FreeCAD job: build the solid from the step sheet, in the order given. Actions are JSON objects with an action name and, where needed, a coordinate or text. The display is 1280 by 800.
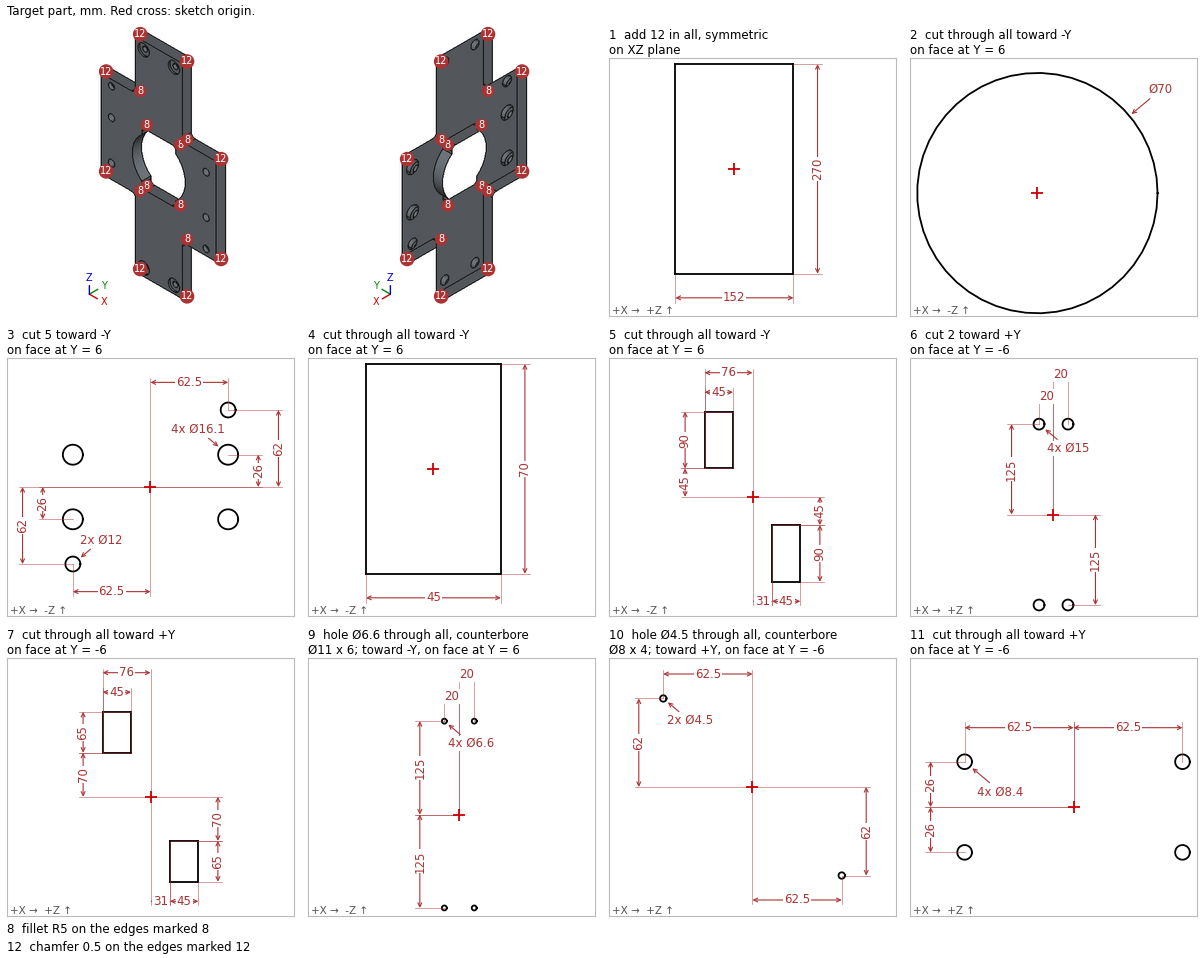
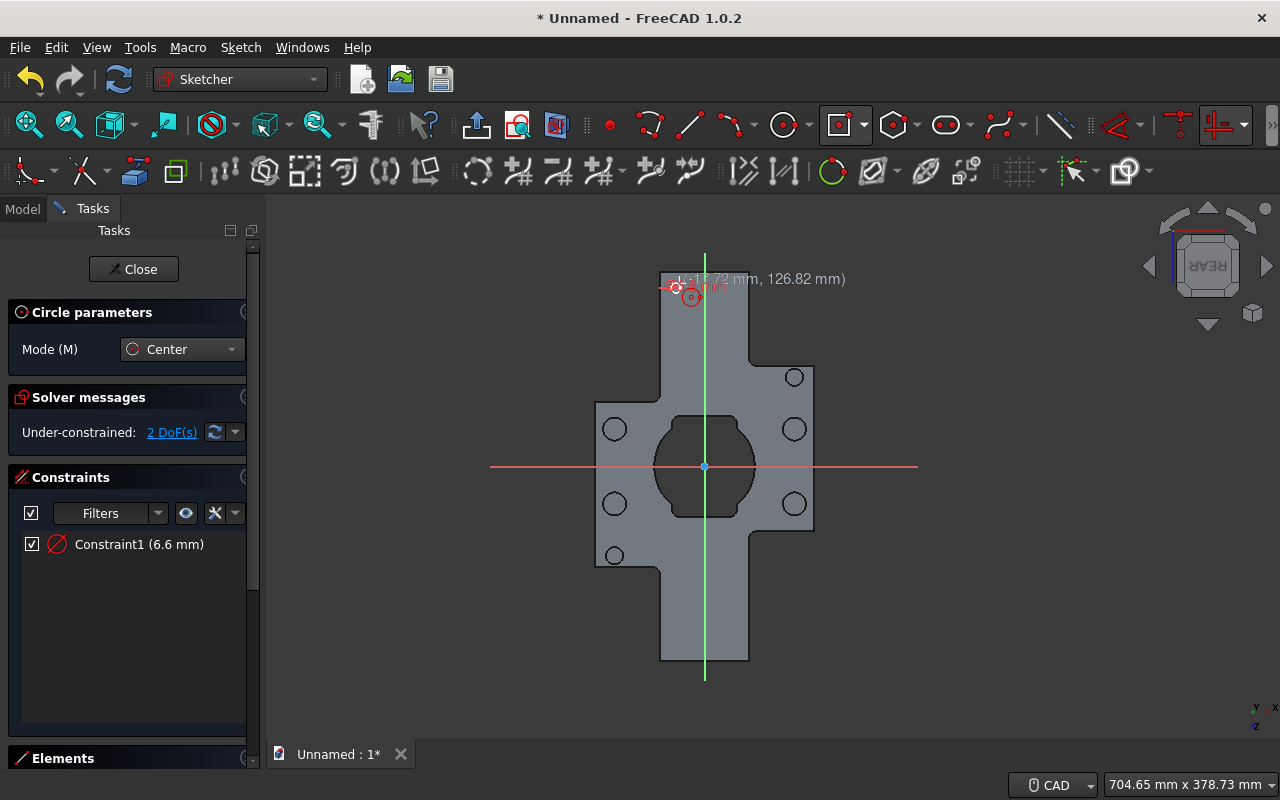
{"action": "scroll", "coordinate": [733, 287], "scroll_direction": "up", "scroll_amount": 8}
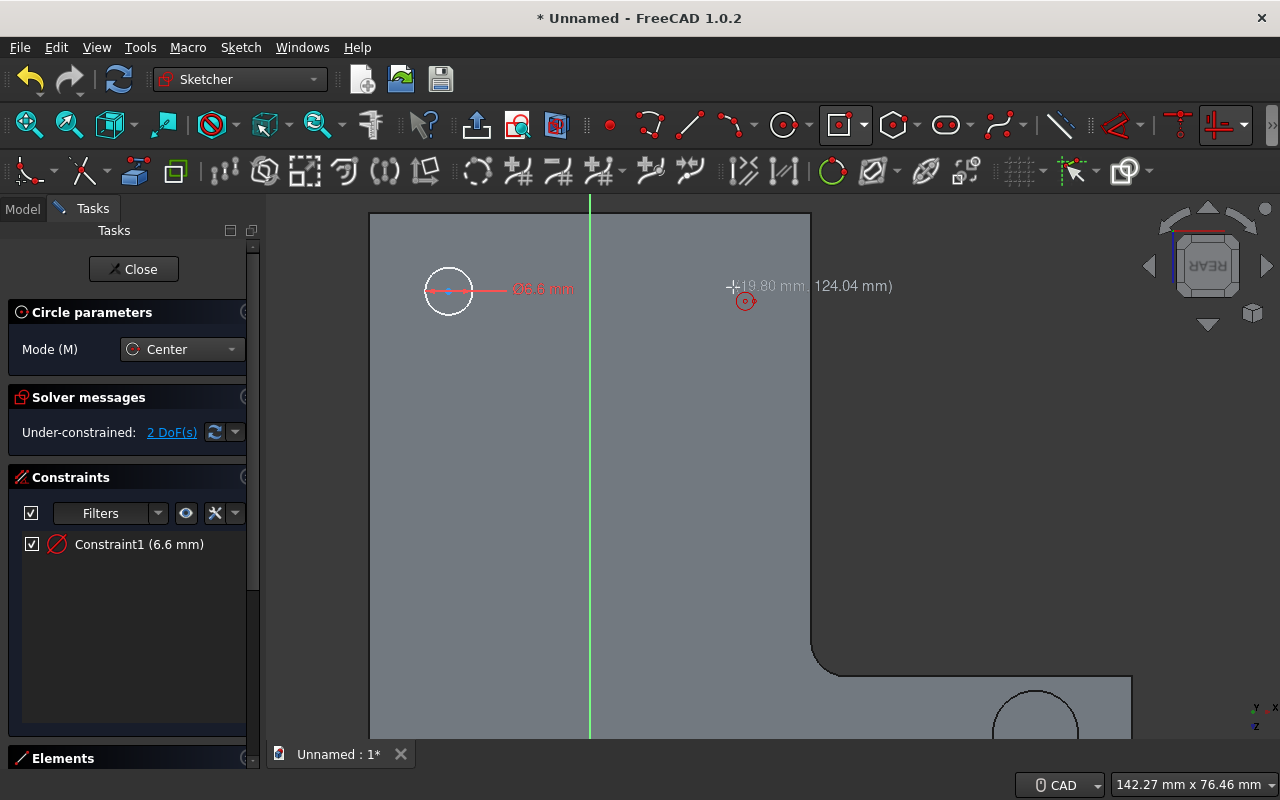
{"action": "scroll", "coordinate": [733, 287], "scroll_direction": "down", "scroll_amount": 8}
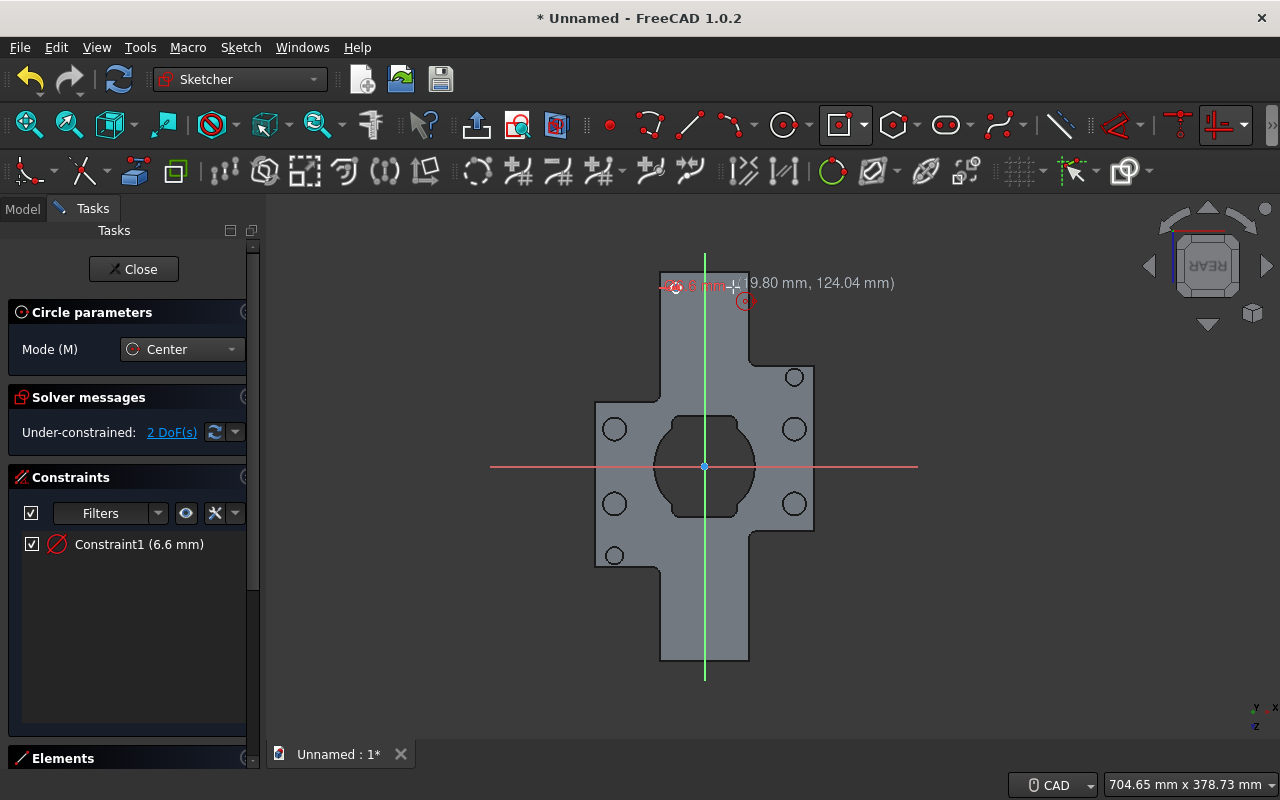
{"action": "left_click", "coordinate": [733, 287]}
{"action": "mouse_move", "coordinate": [737, 283]}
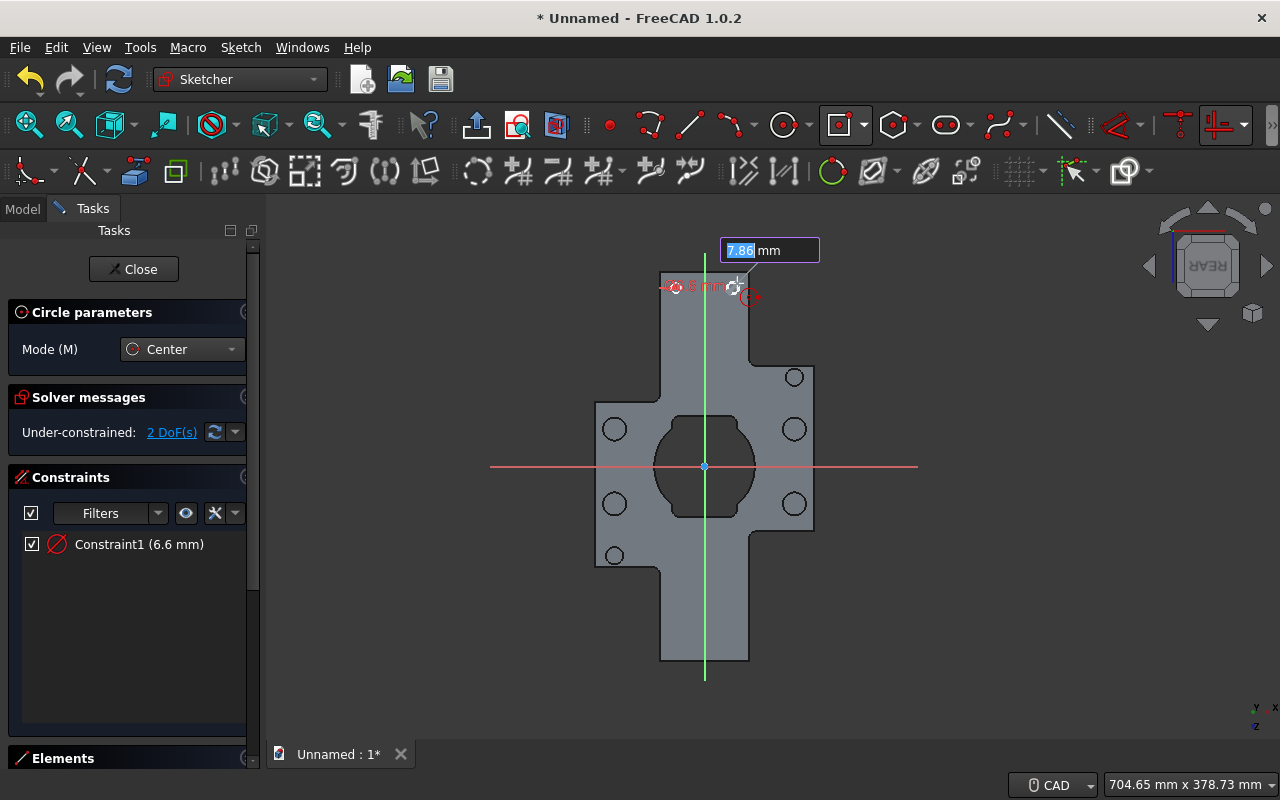
{"action": "type", "text": "6.6"}
{"action": "key", "text": "Return"}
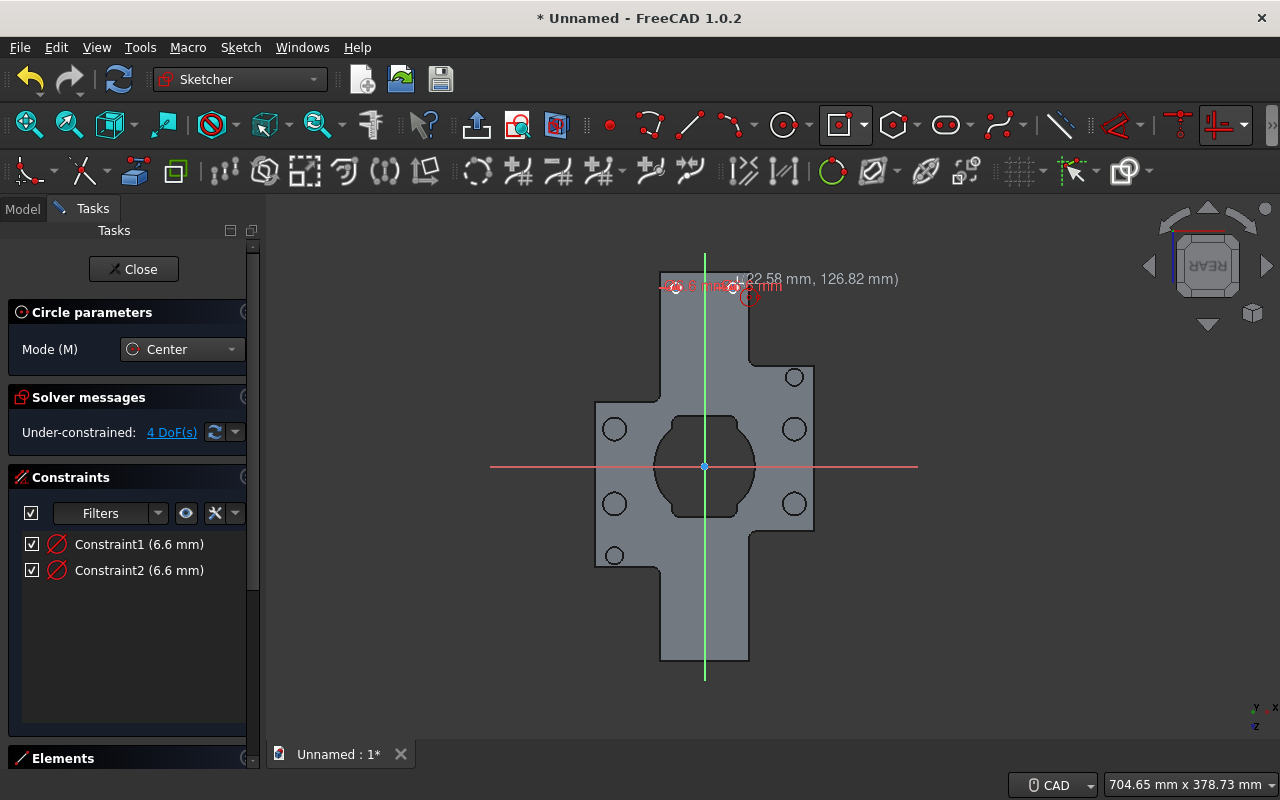
{"action": "scroll", "coordinate": [676, 646], "scroll_direction": "up", "scroll_amount": 8}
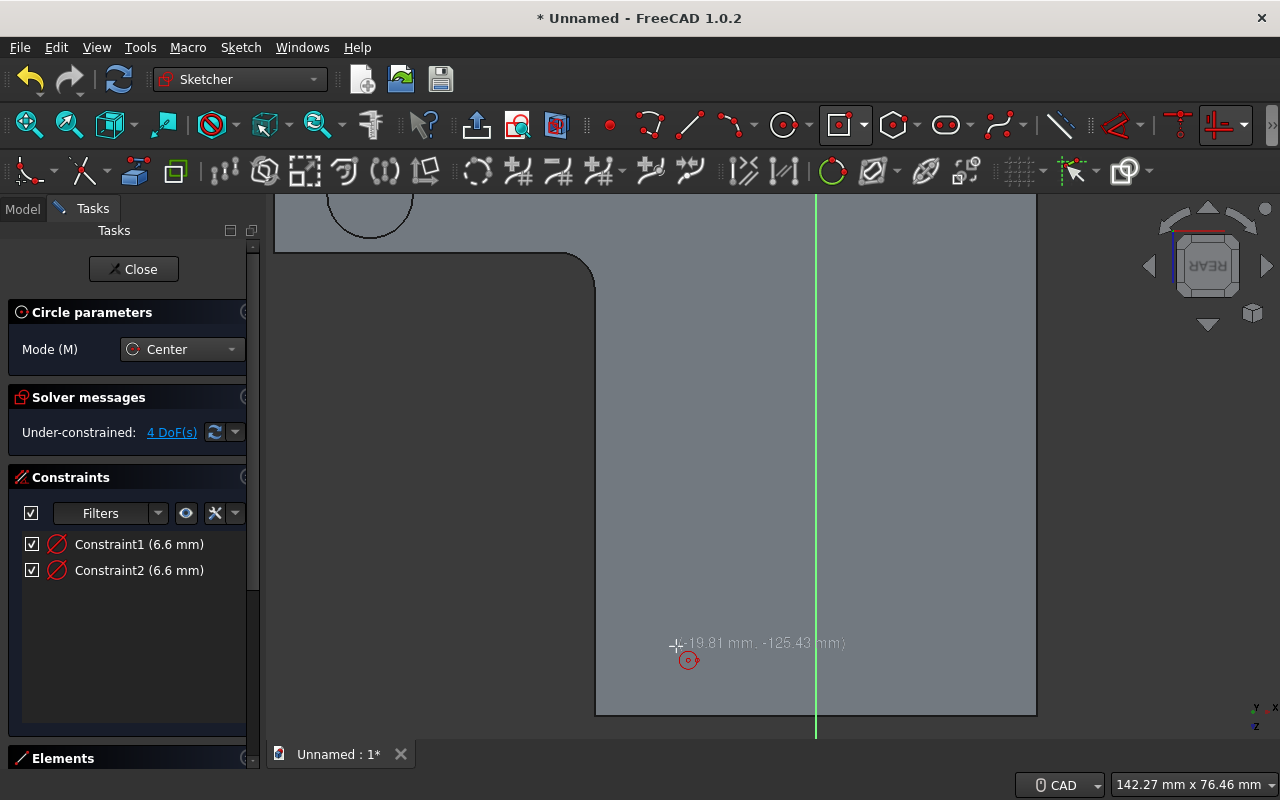
{"action": "scroll", "coordinate": [676, 647], "scroll_direction": "down", "scroll_amount": 8}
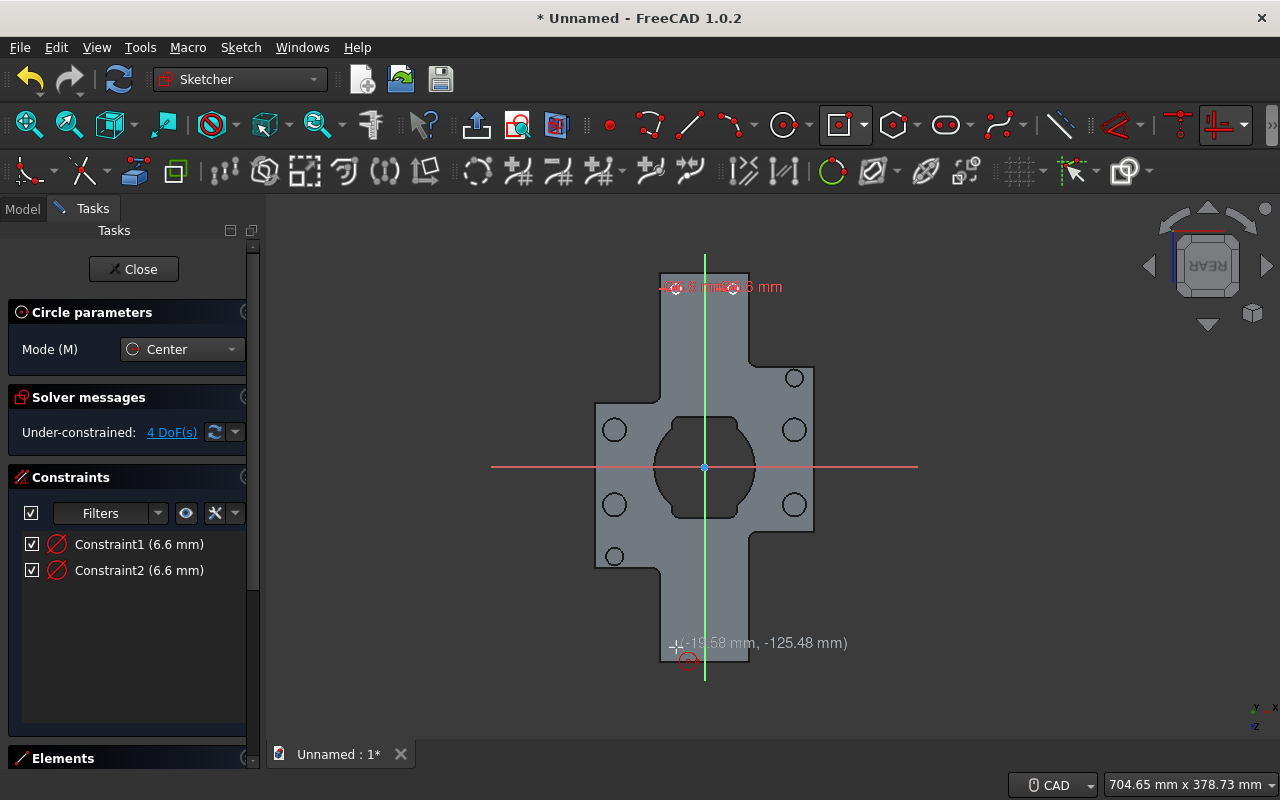
{"action": "left_click", "coordinate": [676, 647]}
{"action": "mouse_move", "coordinate": [679, 644]}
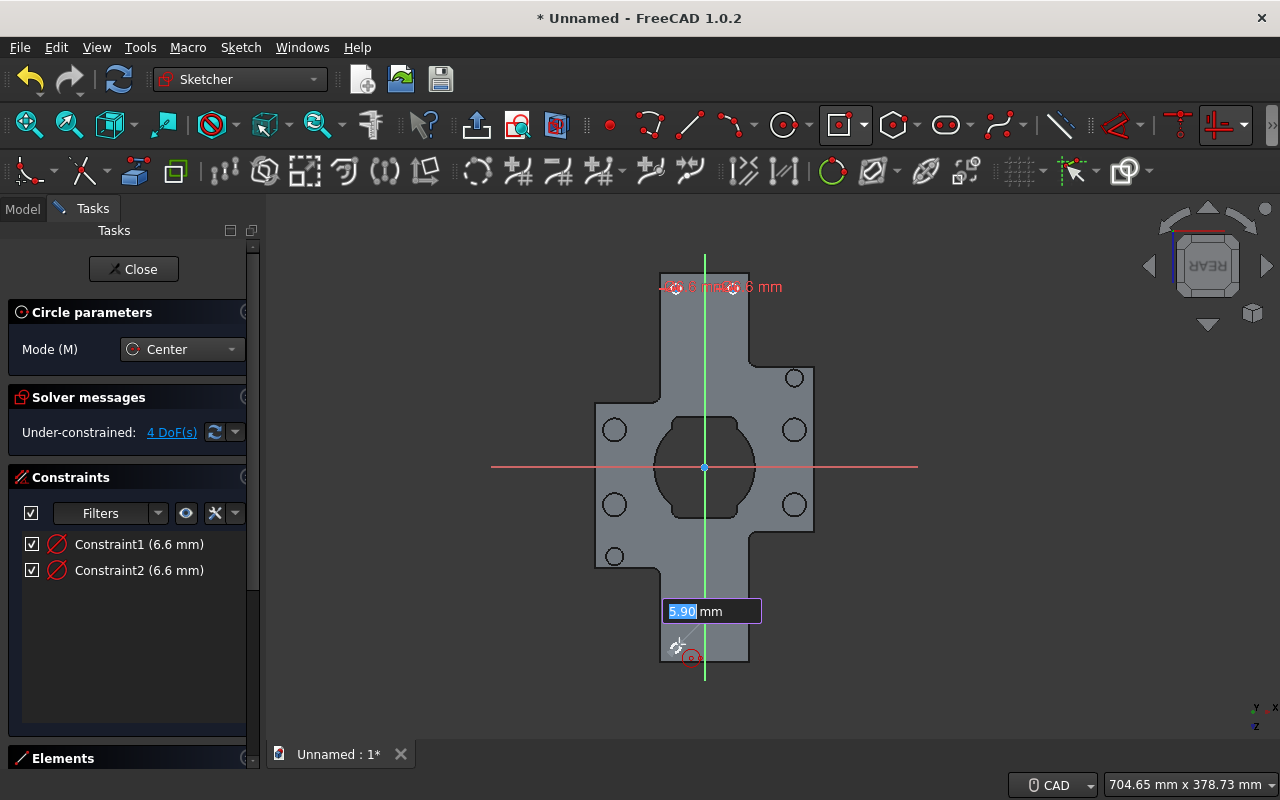
{"action": "type", "text": "6.6"}
{"action": "key", "text": "Return"}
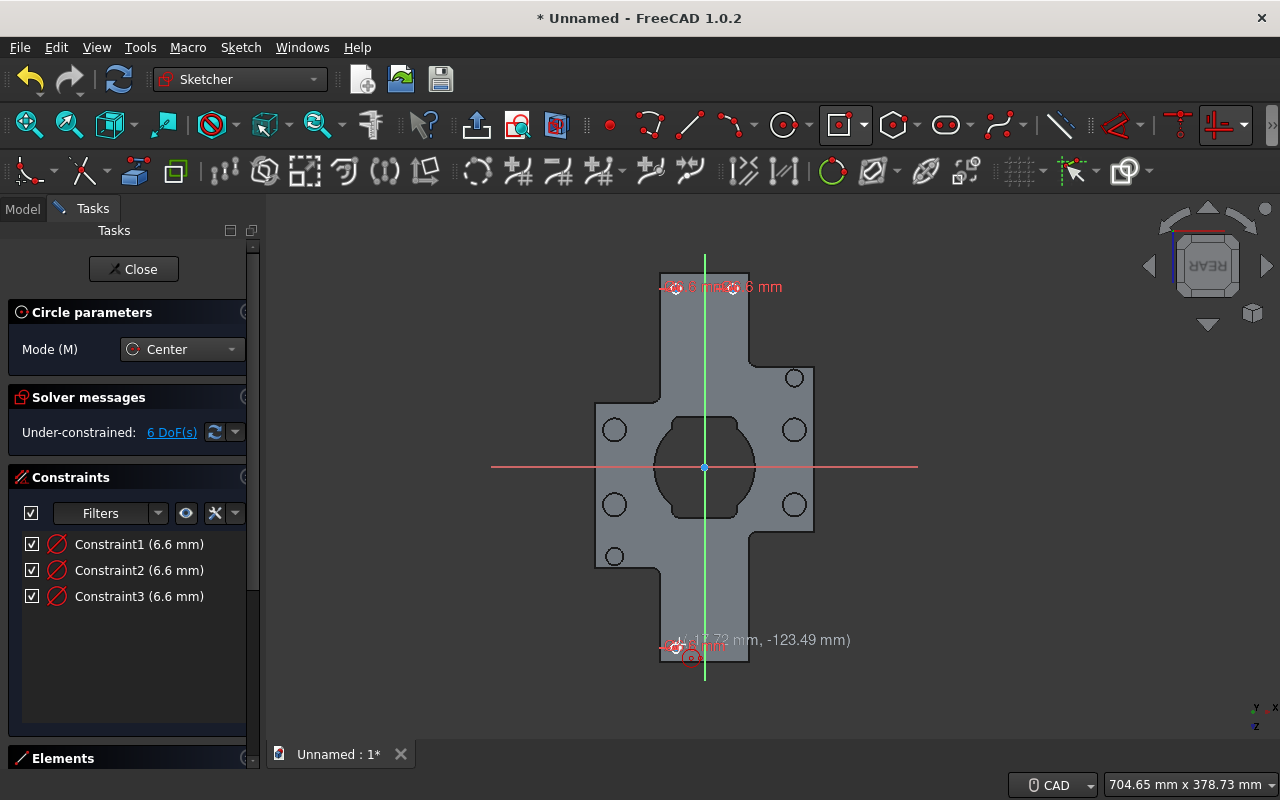
{"action": "scroll", "coordinate": [733, 647], "scroll_direction": "up", "scroll_amount": 8}